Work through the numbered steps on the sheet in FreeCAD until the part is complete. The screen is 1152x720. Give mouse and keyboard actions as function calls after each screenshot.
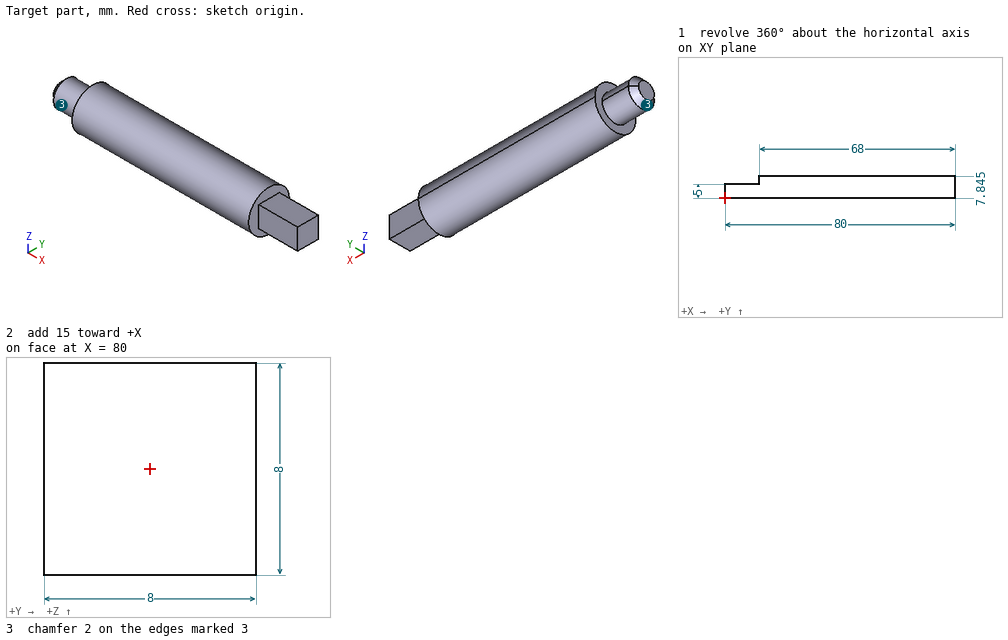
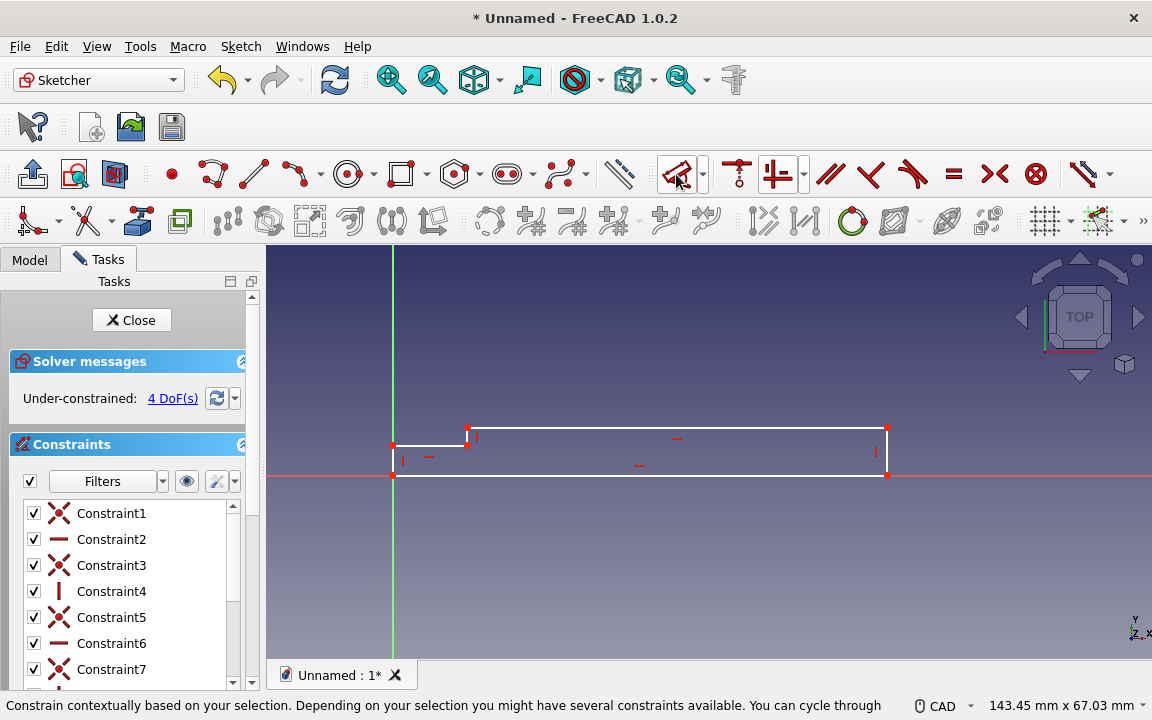
scroll(393, 458, up, 2)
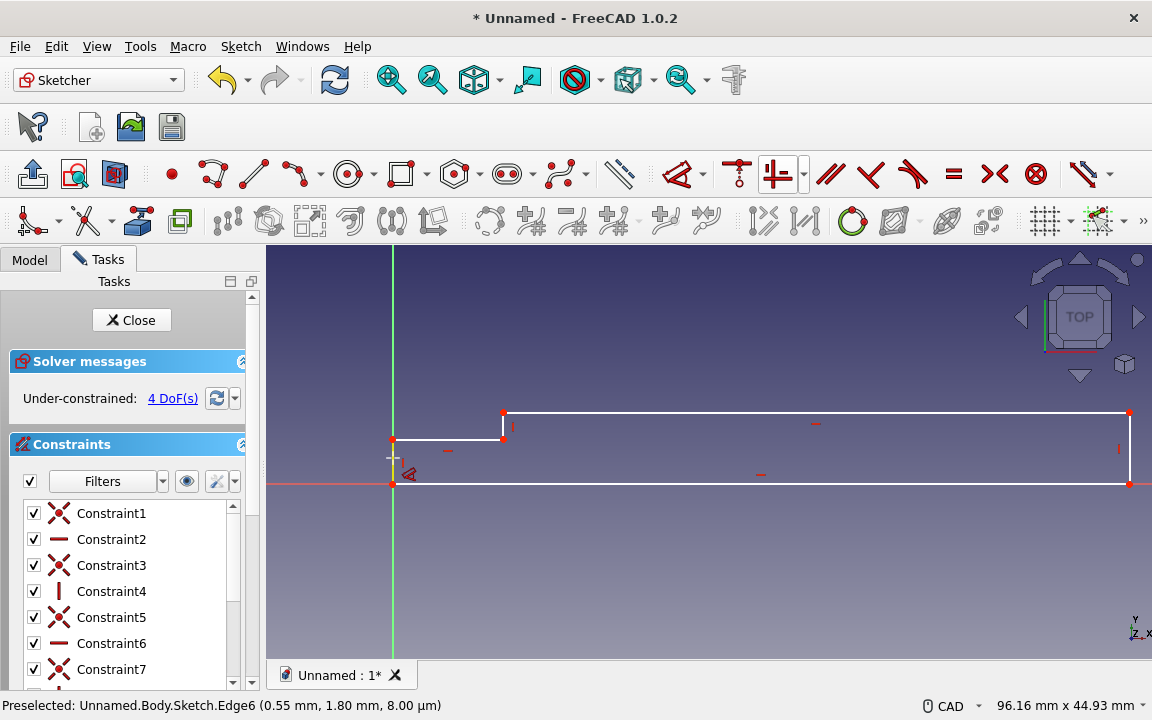
click(393, 458)
click(359, 462)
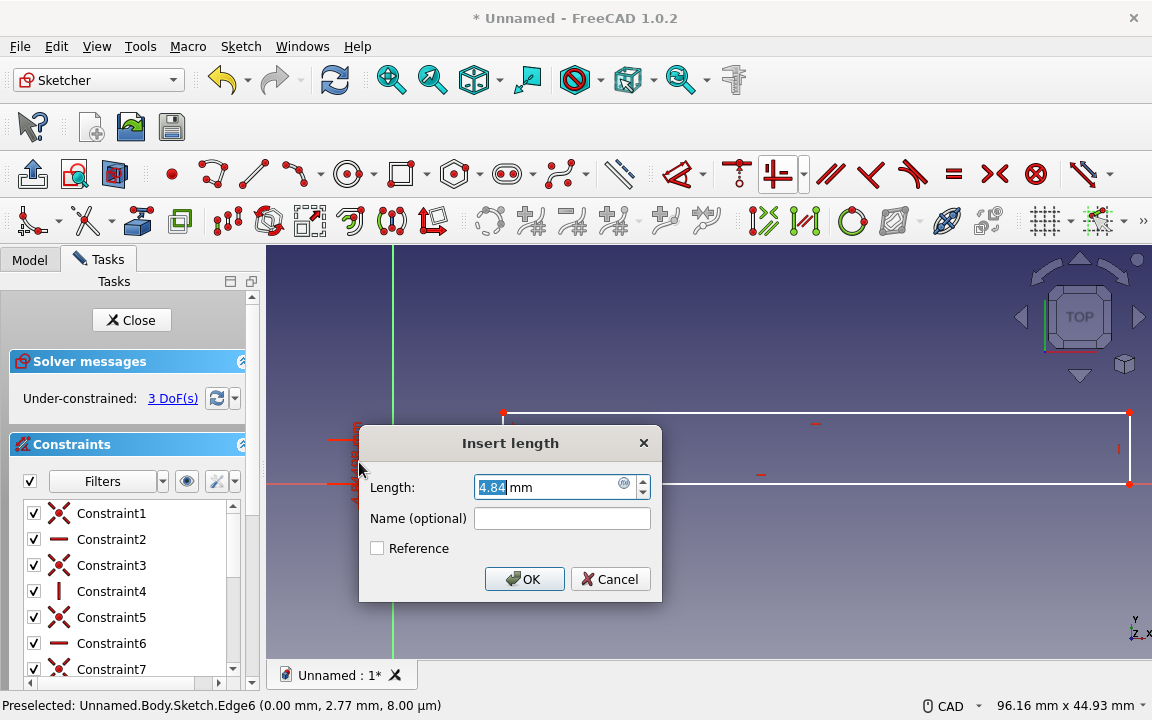
text(5)
key(Return)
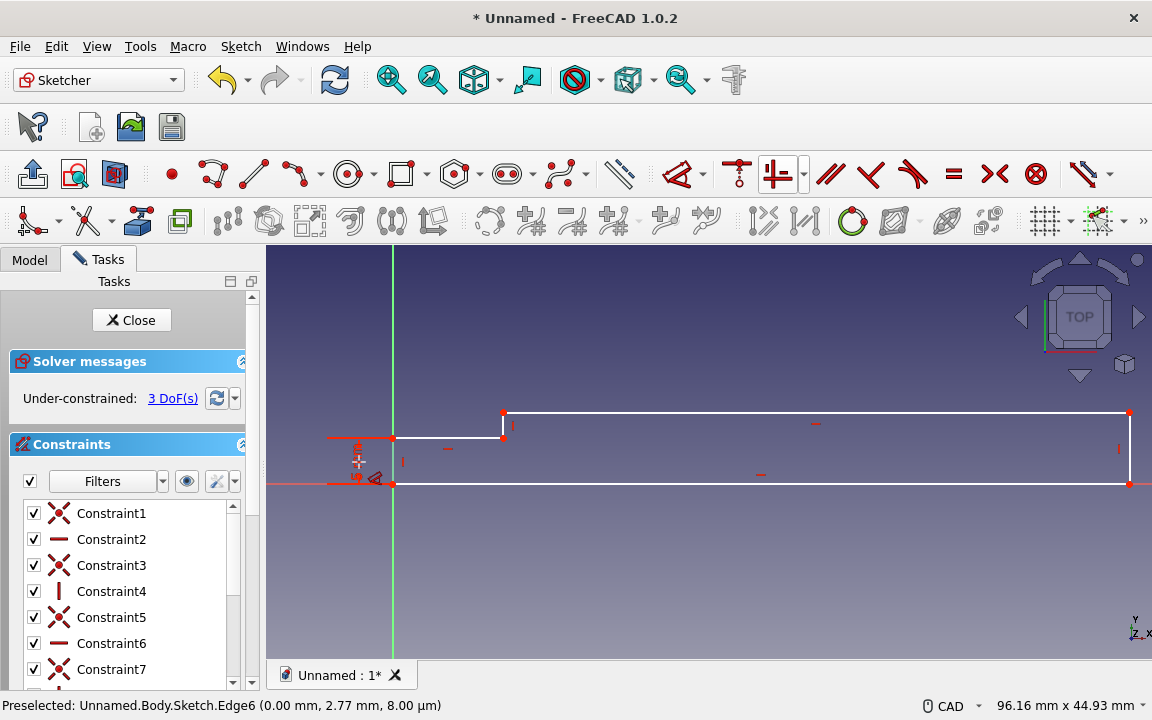
click(614, 484)
click(690, 518)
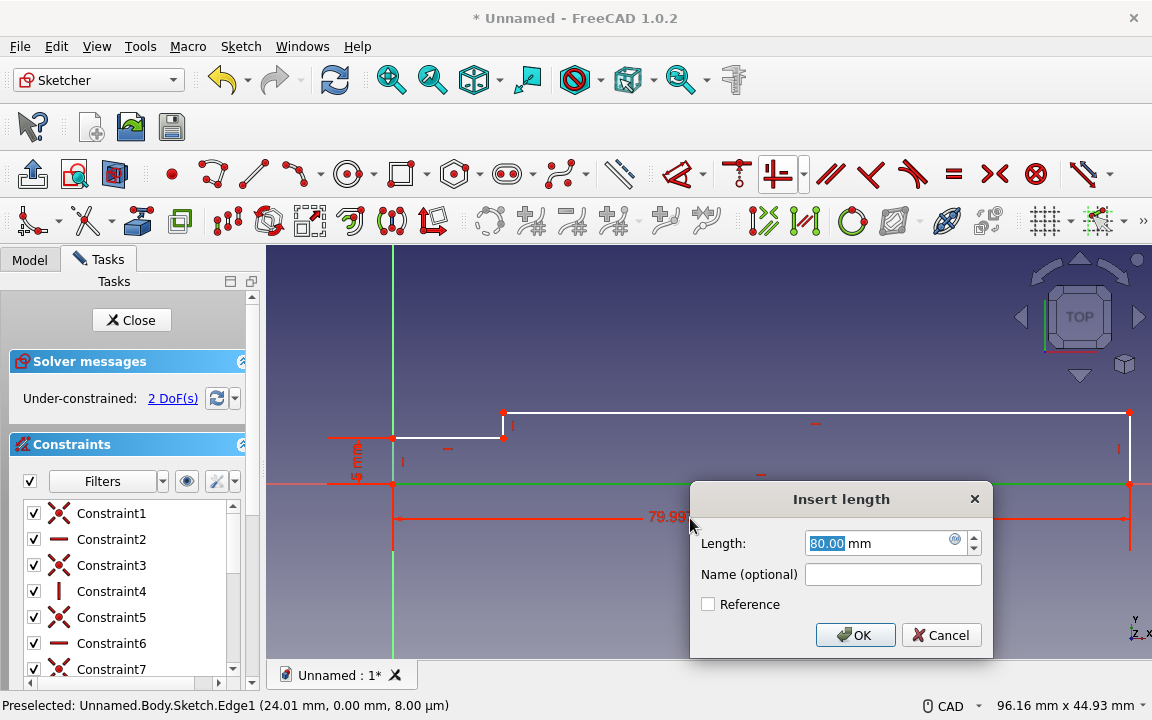
text(80)
key(Return)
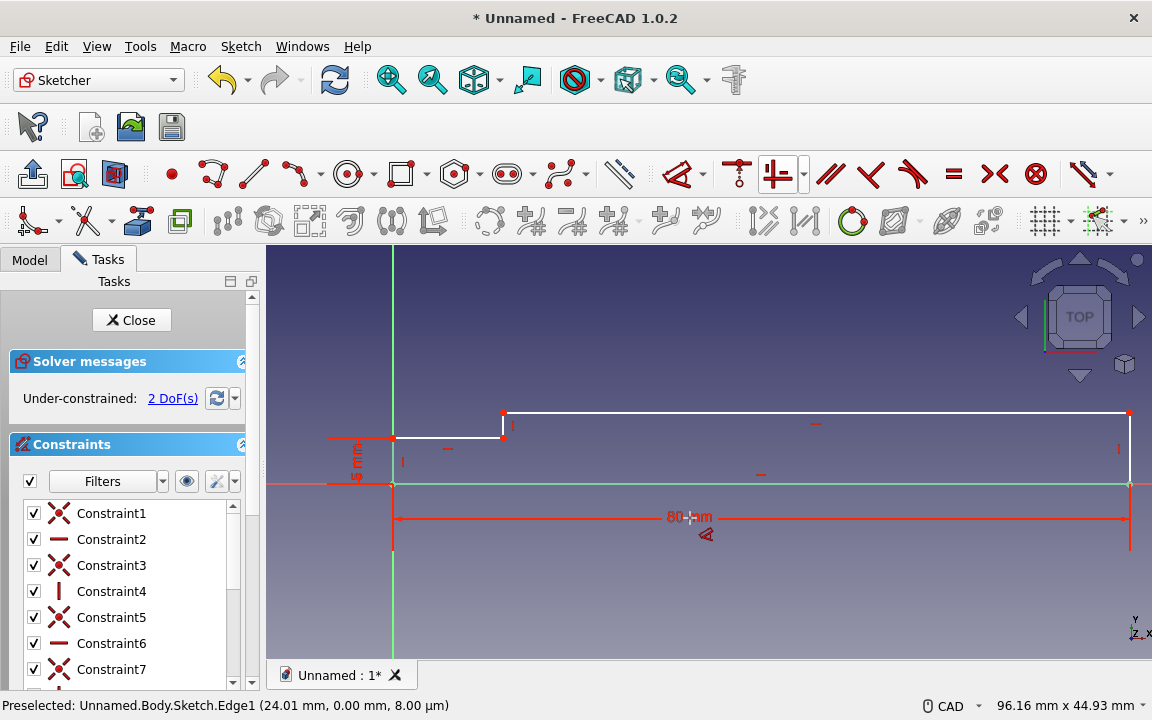
click(942, 413)
click(745, 379)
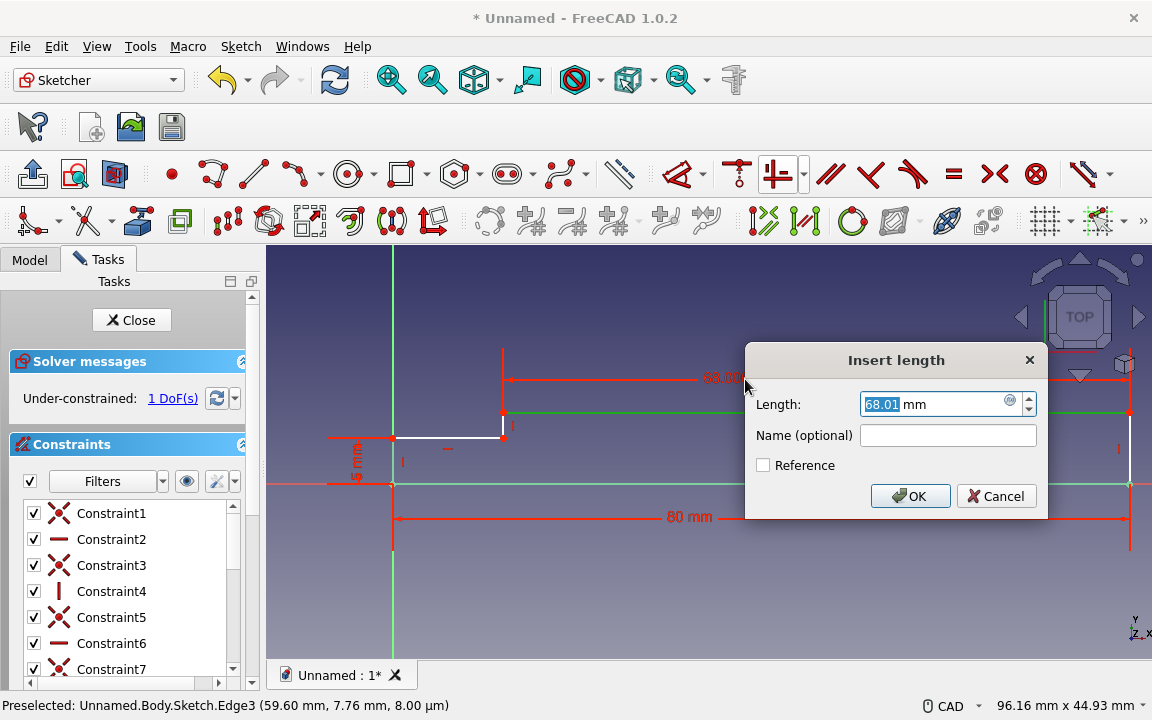
text(68)
key(Return)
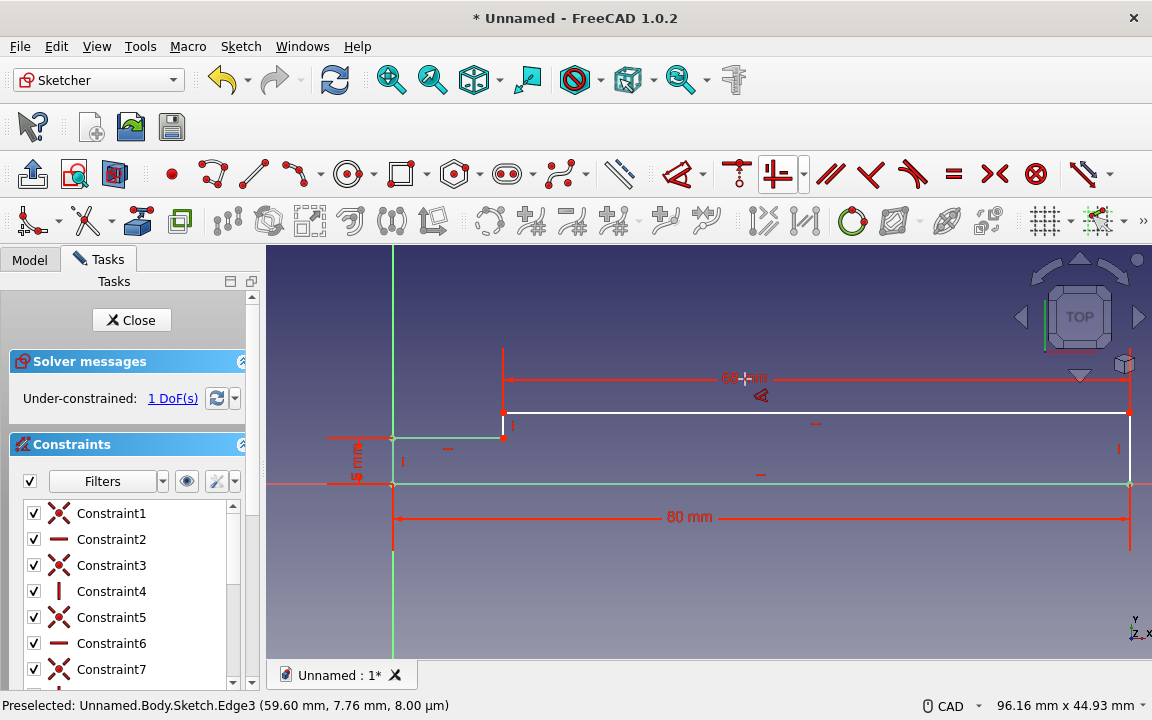
scroll(395, 459, down, 2)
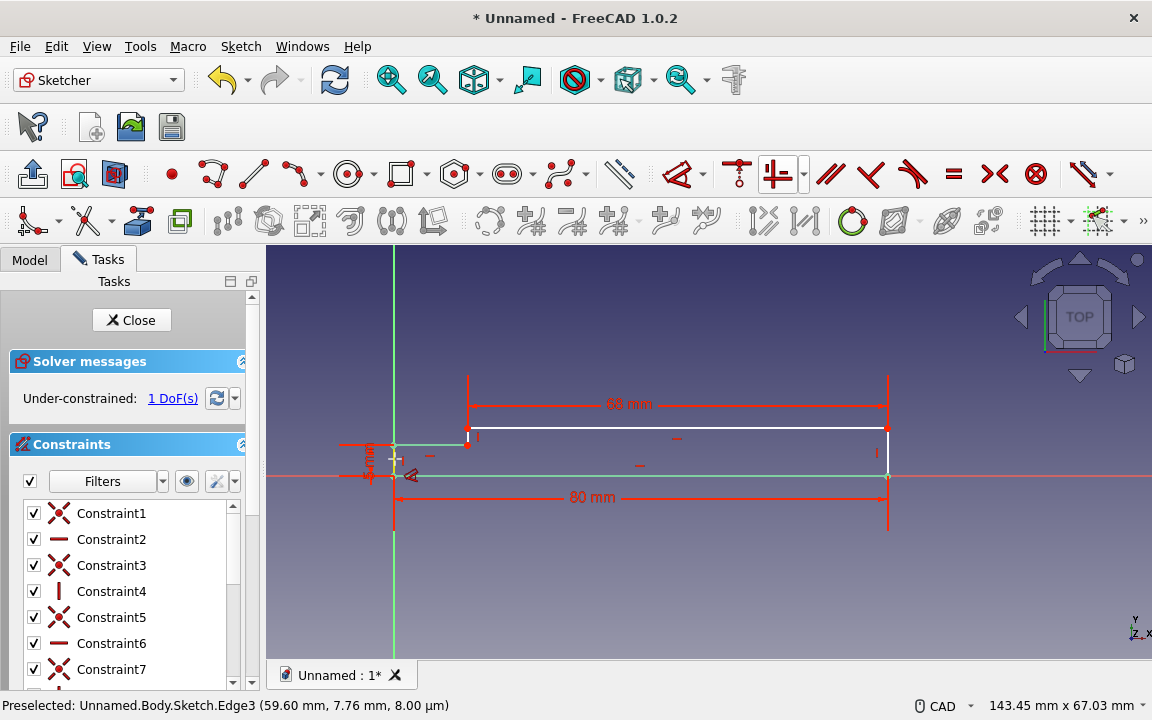
click(888, 462)
click(922, 452)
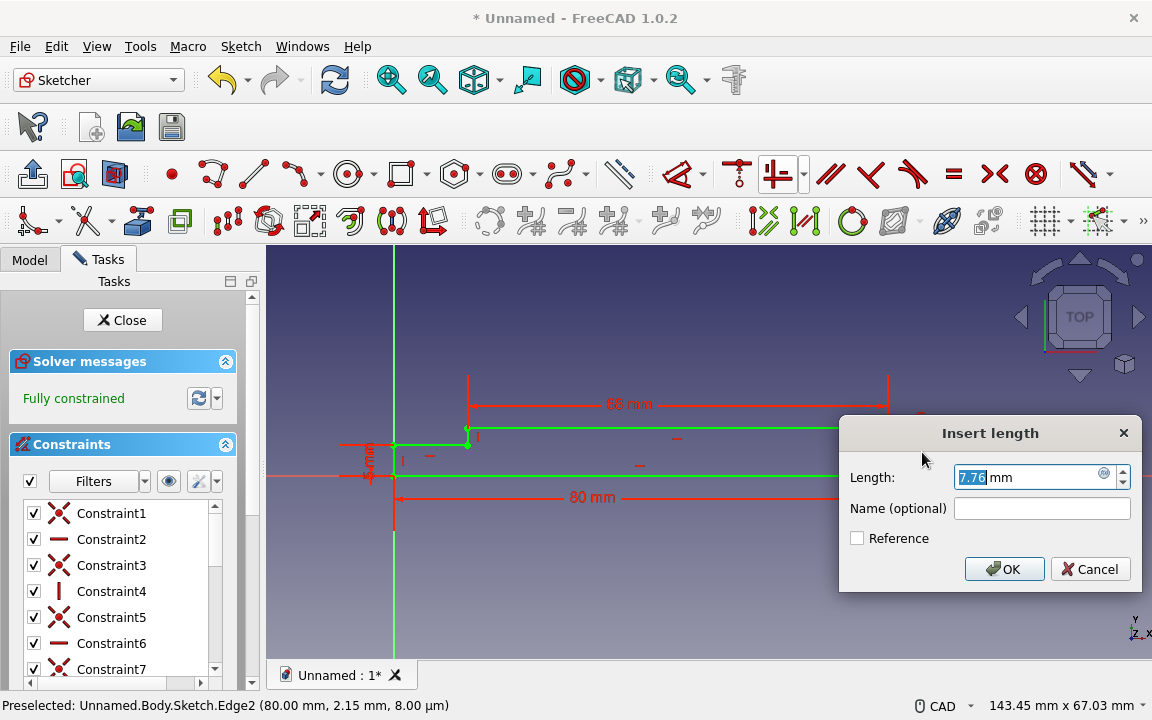
text(7.845)
key(Return)
key(Escape)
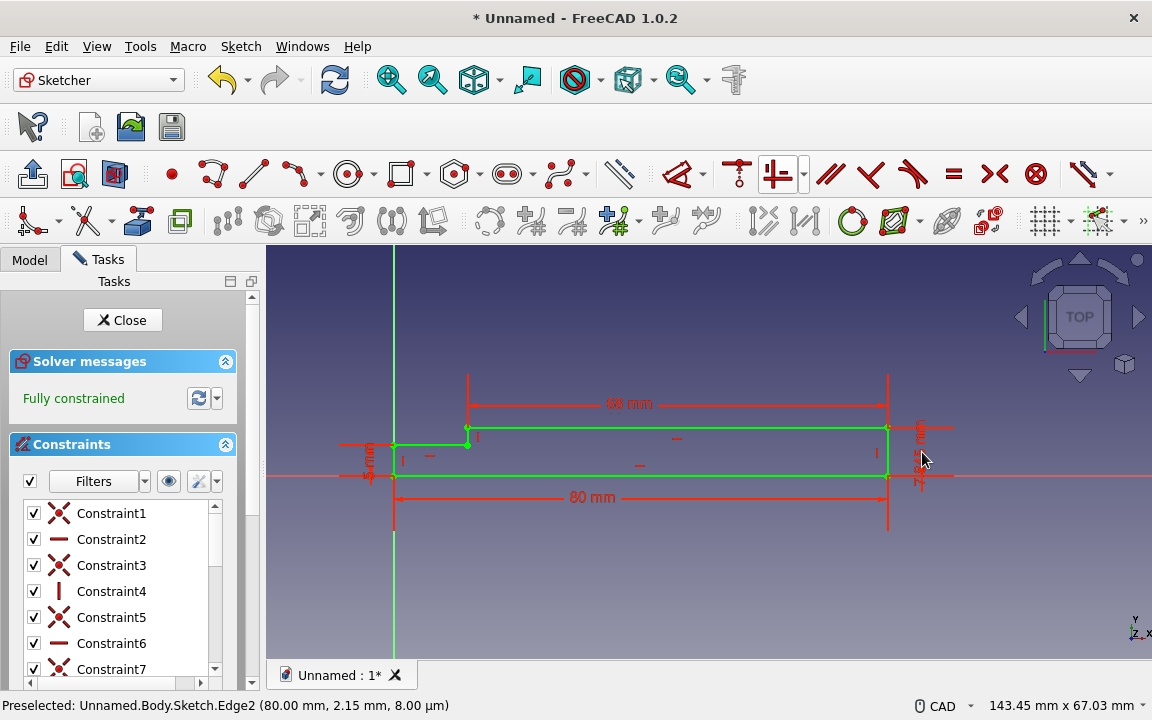
click(123, 320)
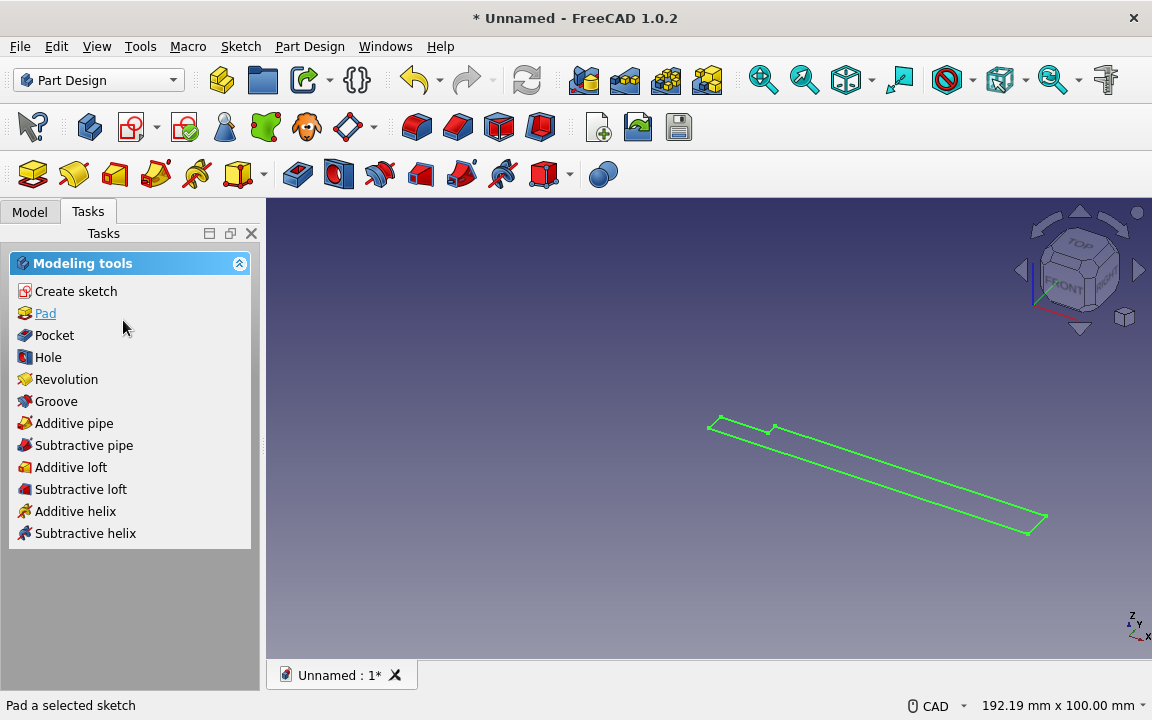
click(74, 174)